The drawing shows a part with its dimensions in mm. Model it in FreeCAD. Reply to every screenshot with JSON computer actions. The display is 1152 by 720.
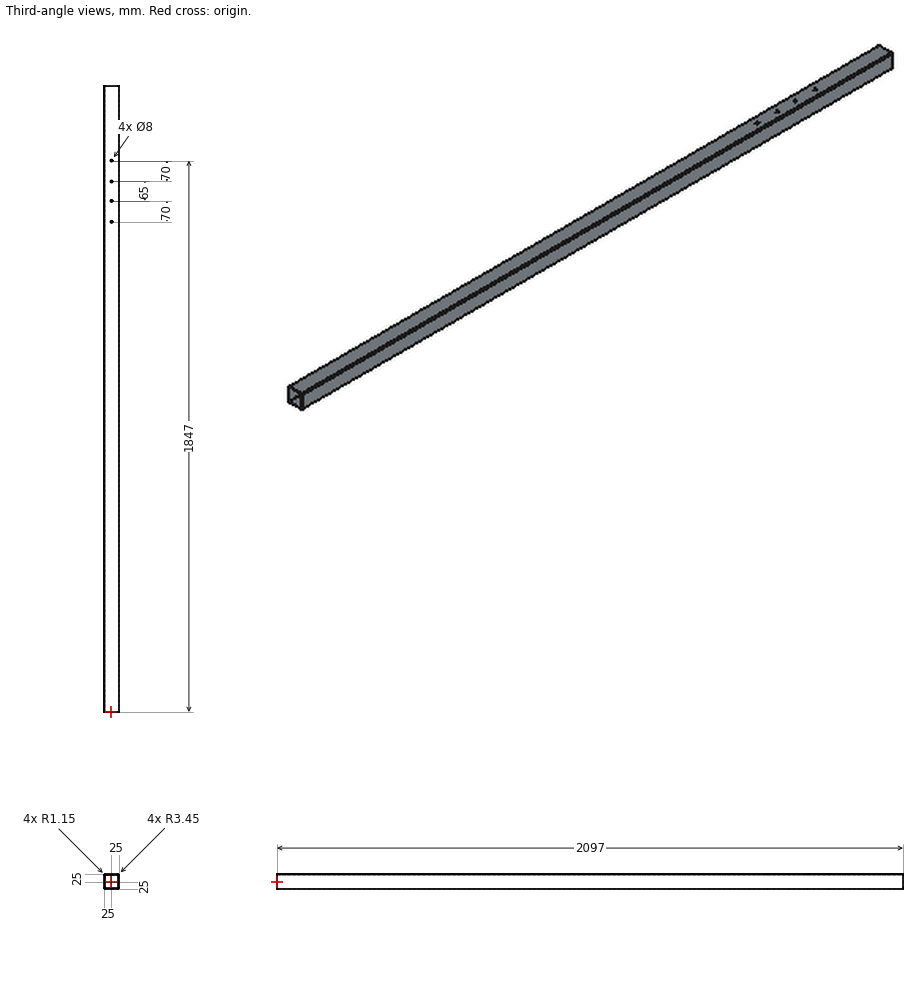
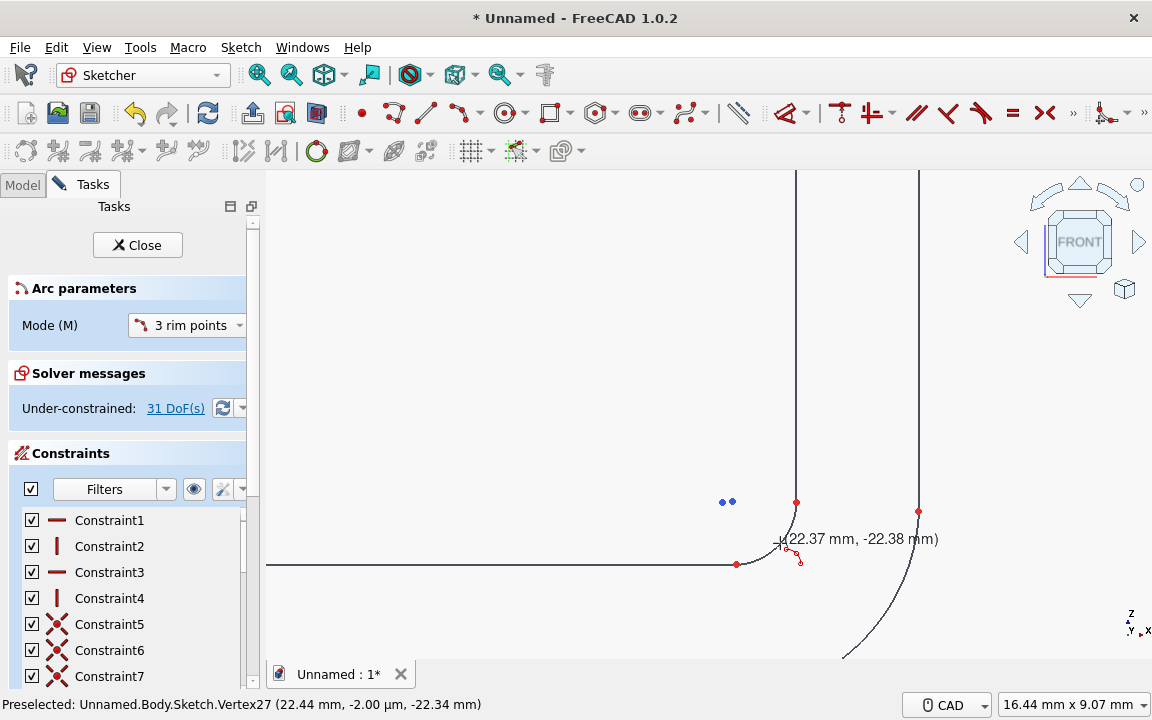
{"action": "scroll", "coordinate": [773, 549], "scroll_direction": "down", "scroll_amount": 11}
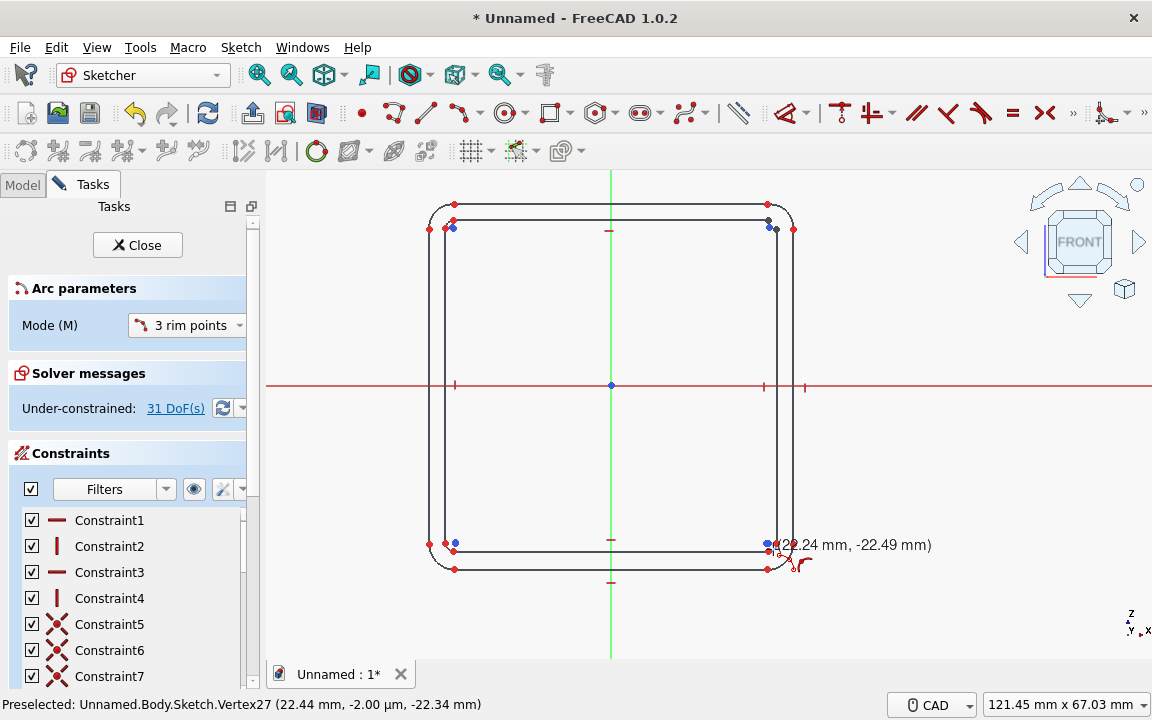
{"action": "scroll", "coordinate": [776, 287], "scroll_direction": "up", "scroll_amount": 5}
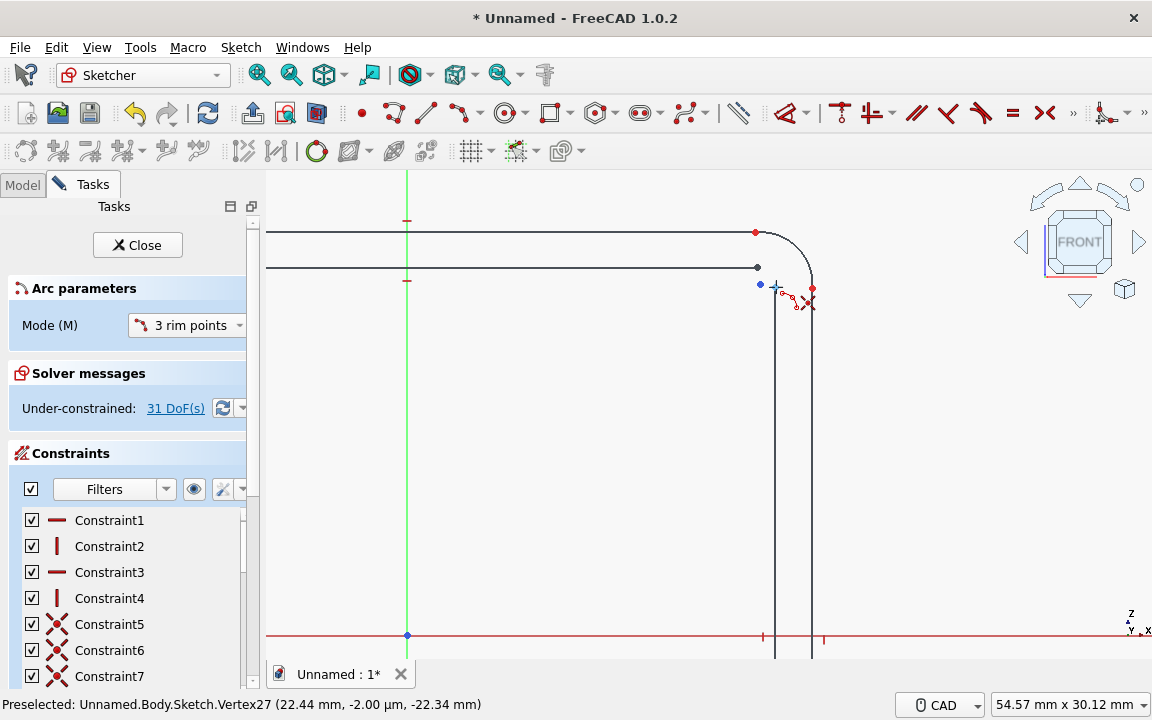
{"action": "left_click", "coordinate": [775, 287]}
{"action": "left_click", "coordinate": [757, 268]}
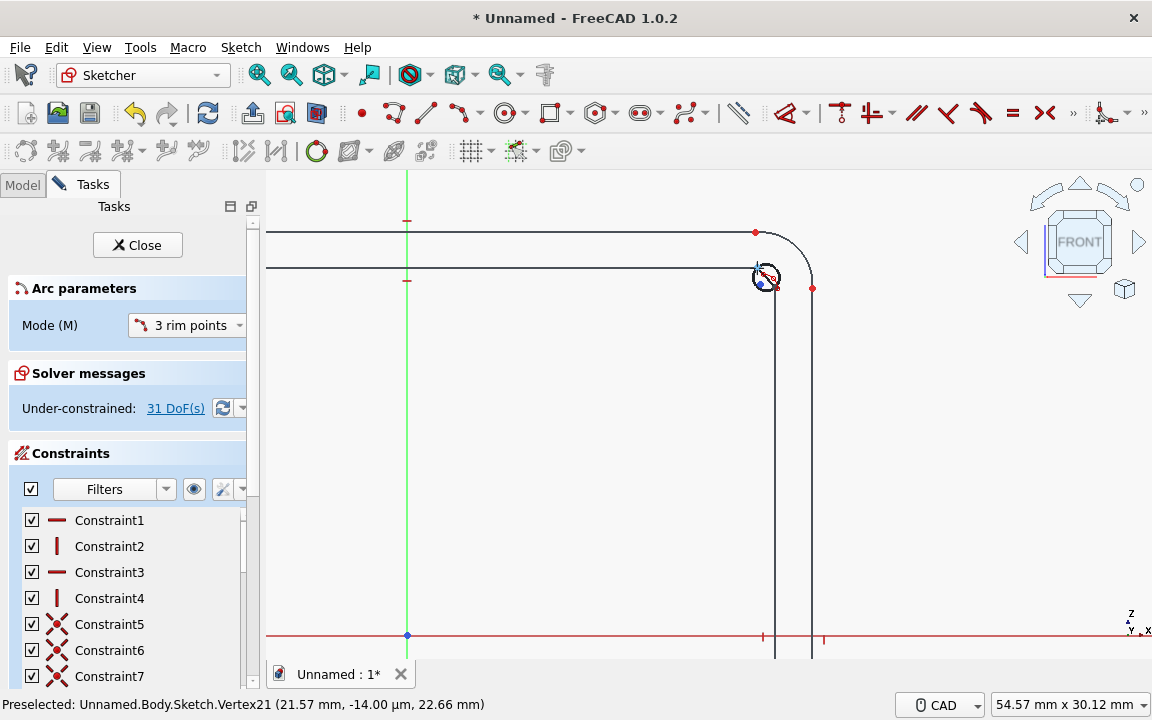
{"action": "scroll", "coordinate": [770, 273], "scroll_direction": "up", "scroll_amount": 6}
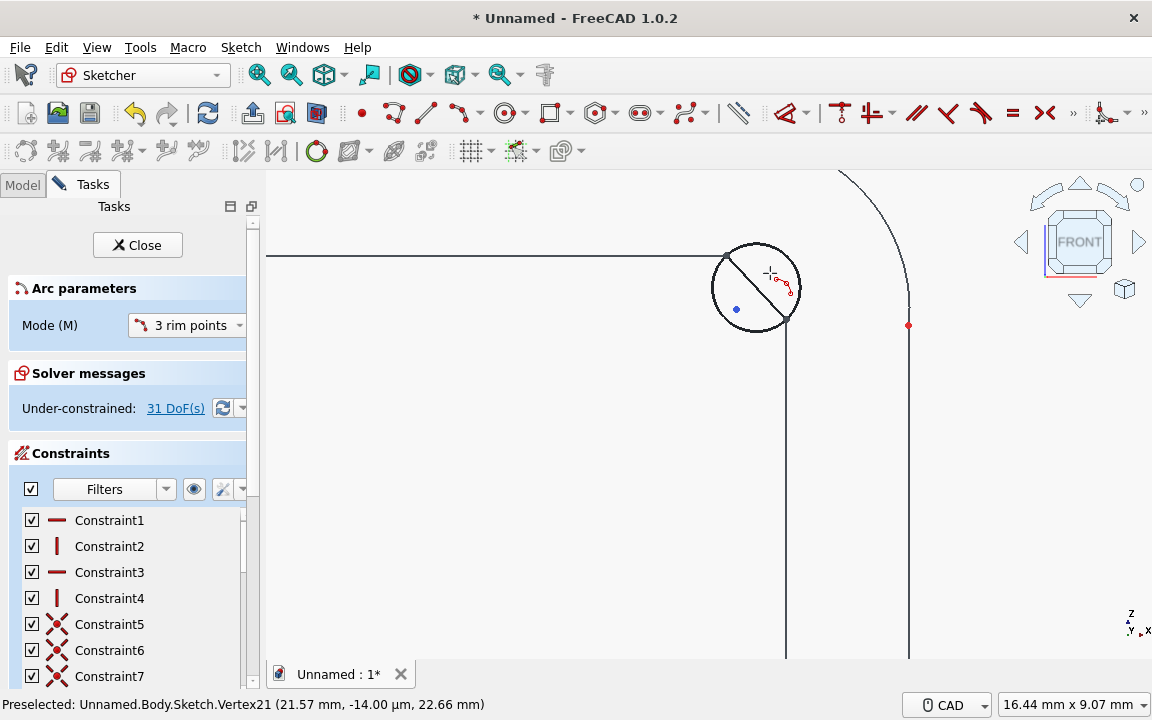
{"action": "left_click", "coordinate": [769, 272]}
{"action": "key", "text": "Escape"}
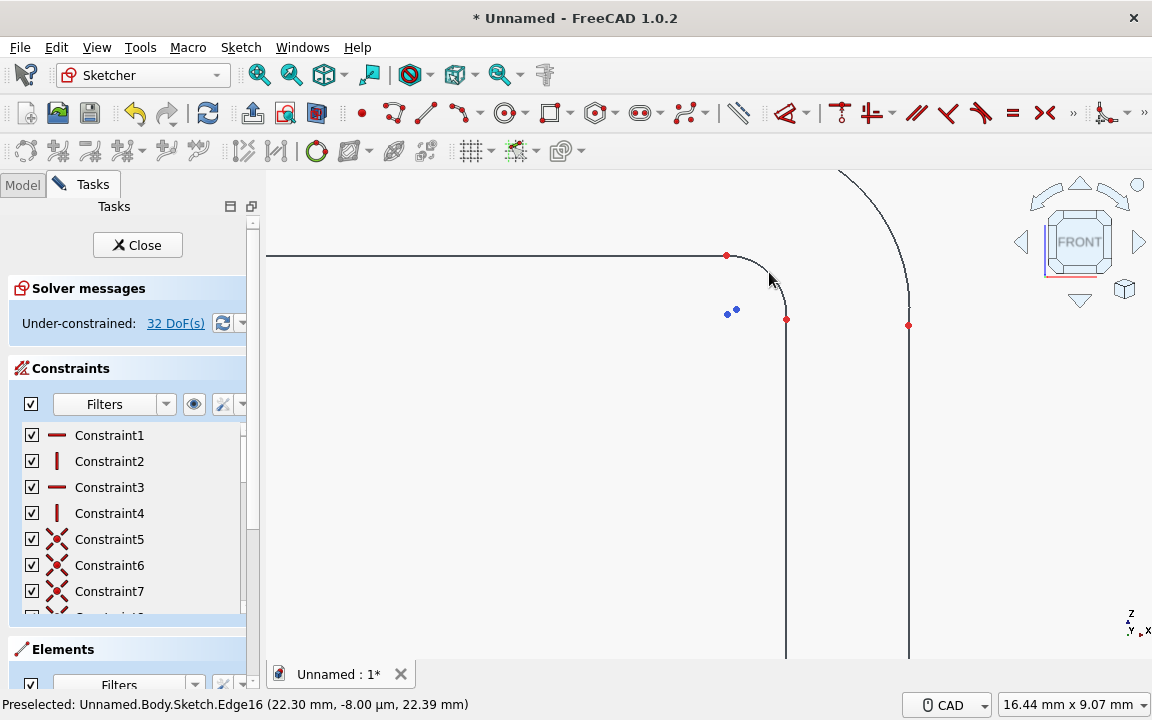
{"action": "scroll", "coordinate": [775, 282], "scroll_direction": "down", "scroll_amount": 11}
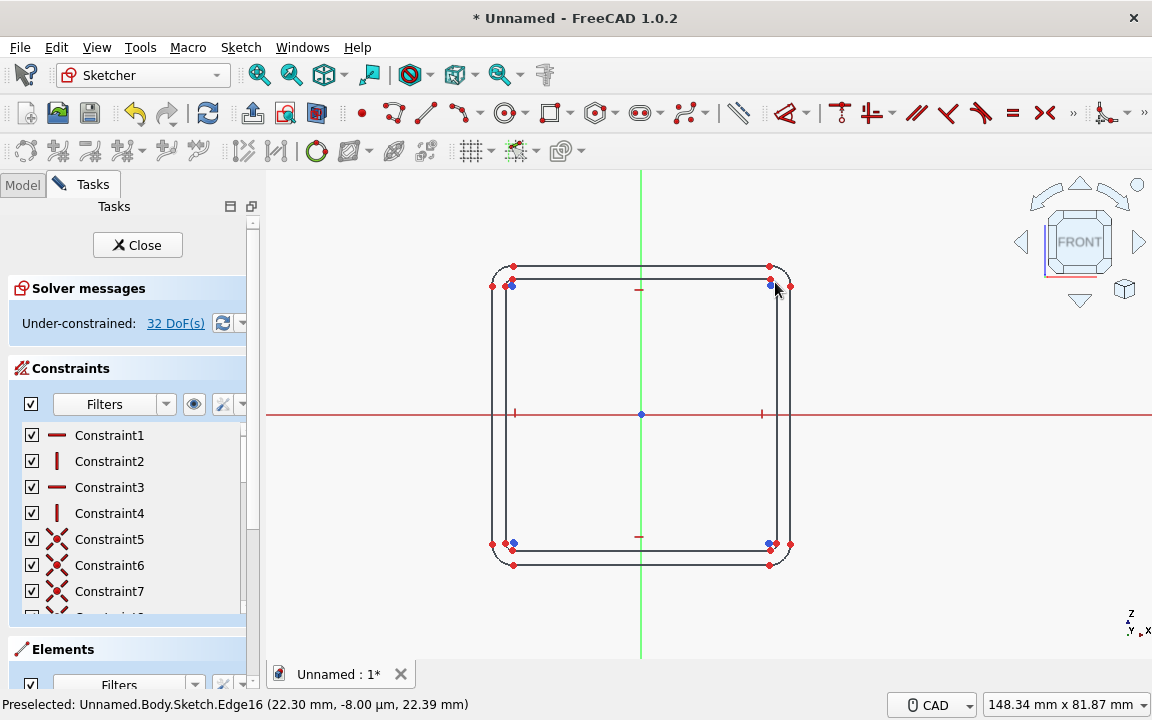
{"action": "left_click", "coordinate": [590, 266]}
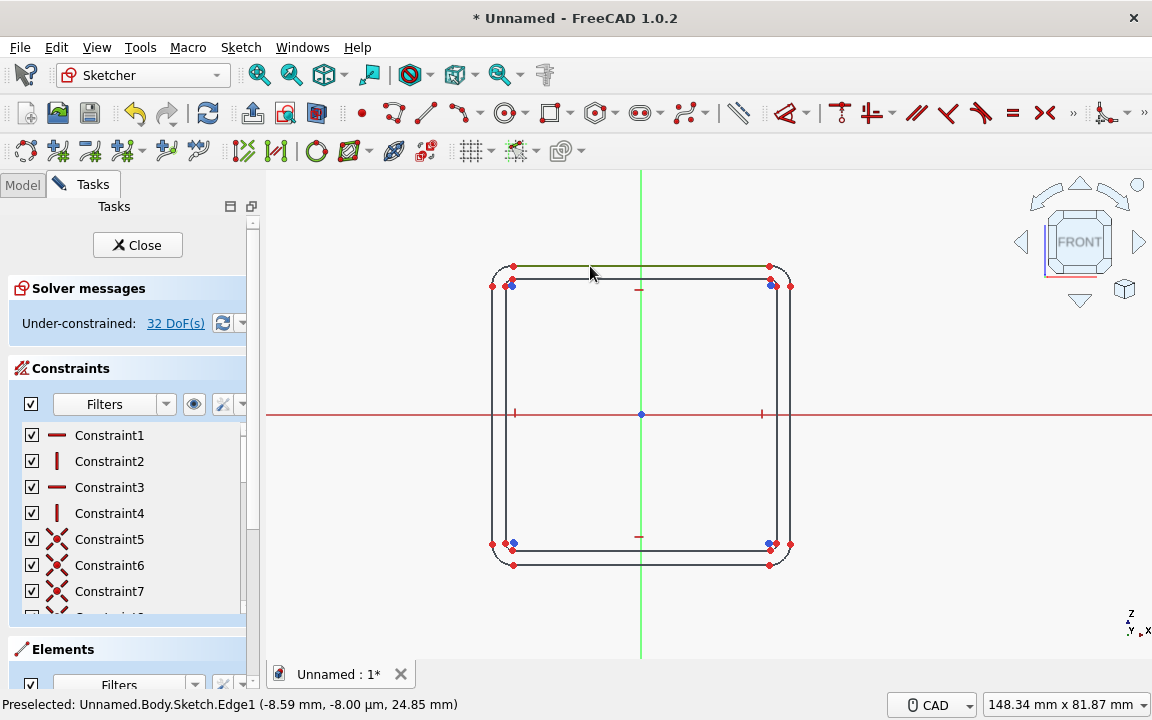
{"action": "scroll", "coordinate": [789, 277], "scroll_direction": "up", "scroll_amount": 2}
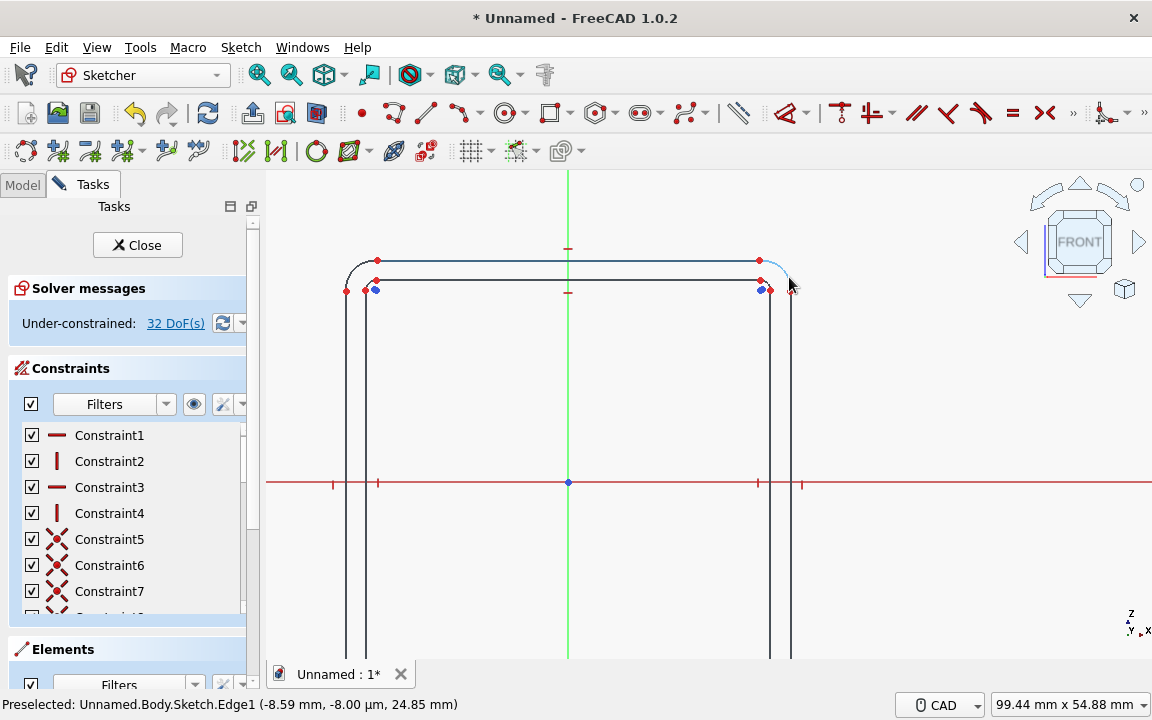
{"action": "left_click", "coordinate": [788, 277]}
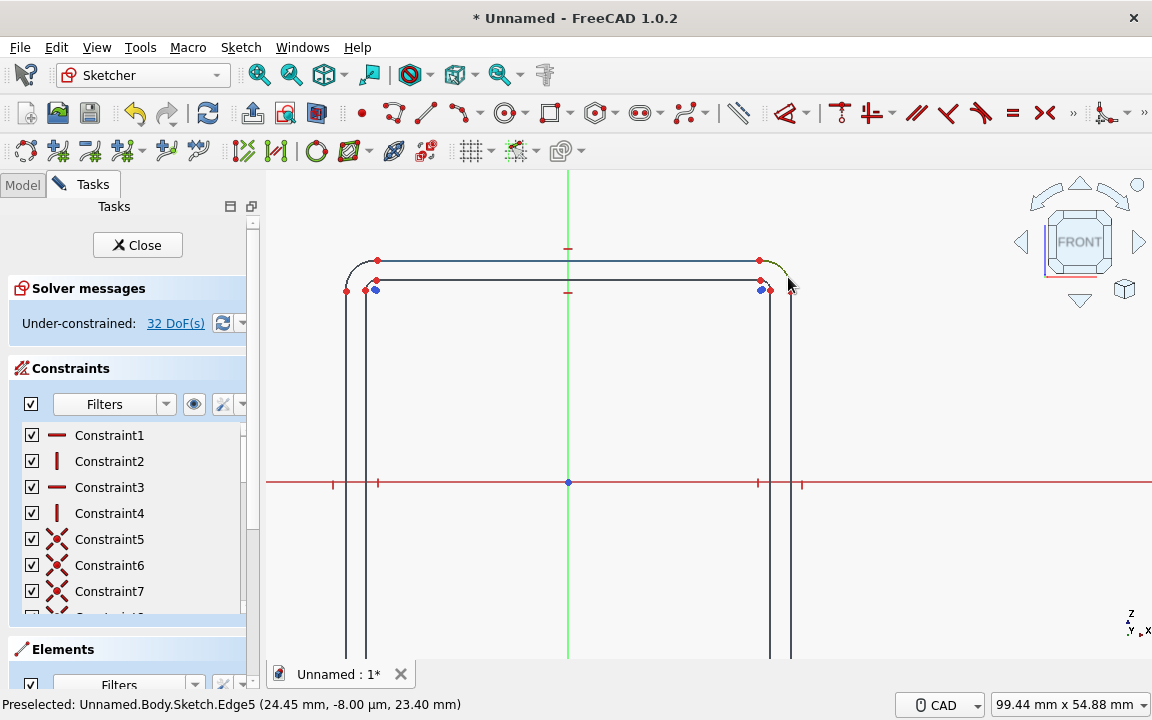
{"action": "left_click", "coordinate": [982, 114]}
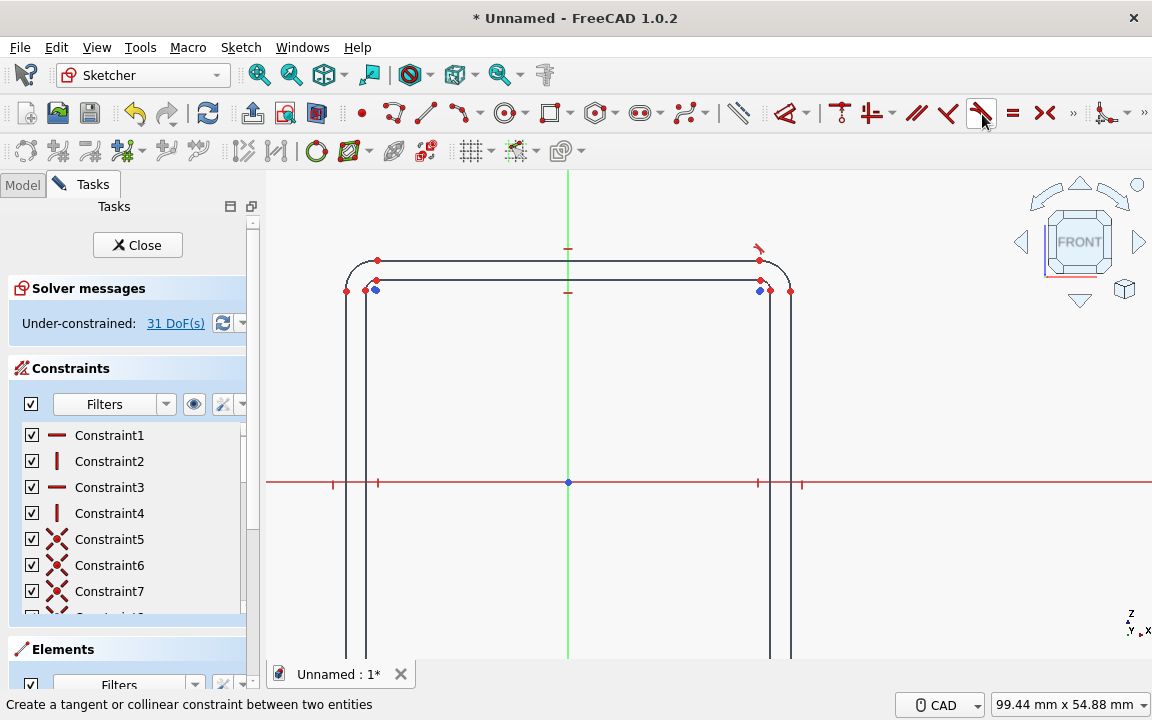
{"action": "left_click", "coordinate": [492, 261]}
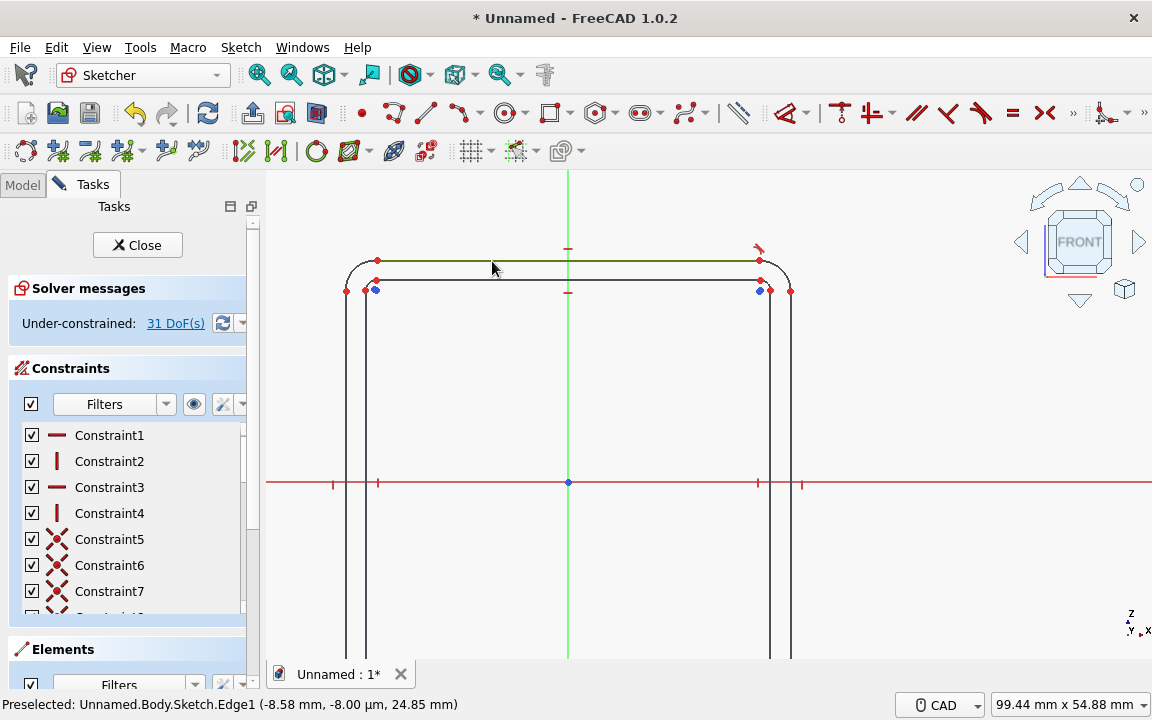
{"action": "left_click", "coordinate": [362, 263]}